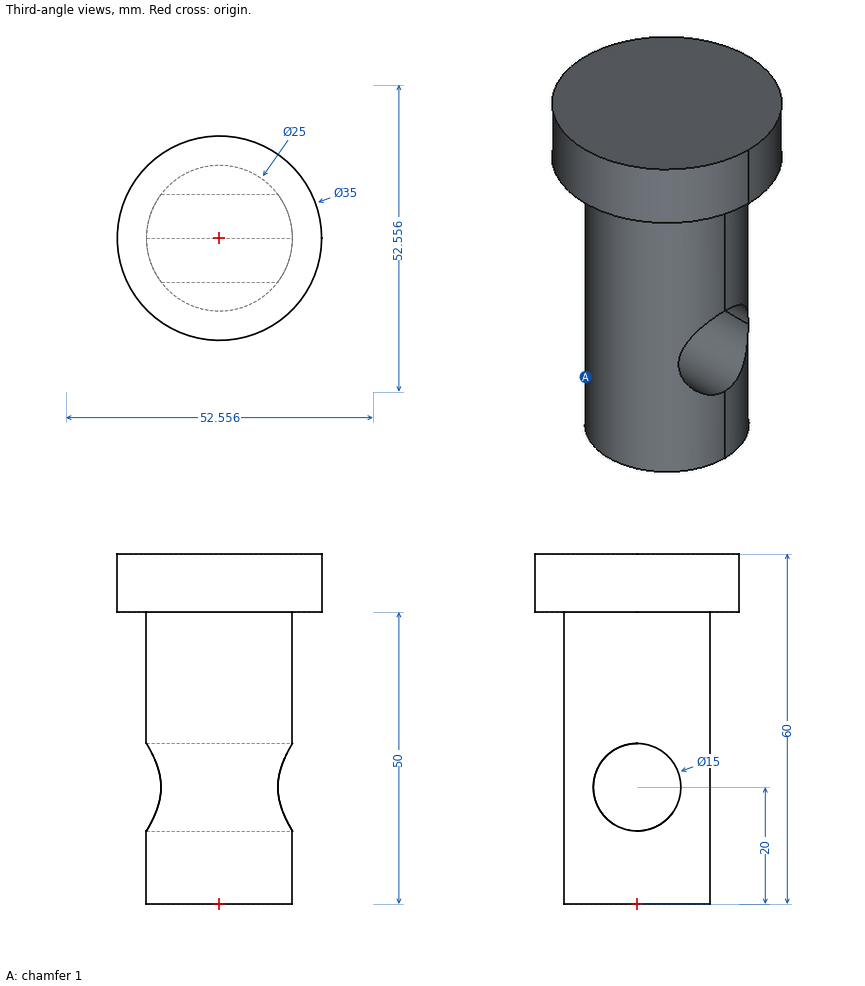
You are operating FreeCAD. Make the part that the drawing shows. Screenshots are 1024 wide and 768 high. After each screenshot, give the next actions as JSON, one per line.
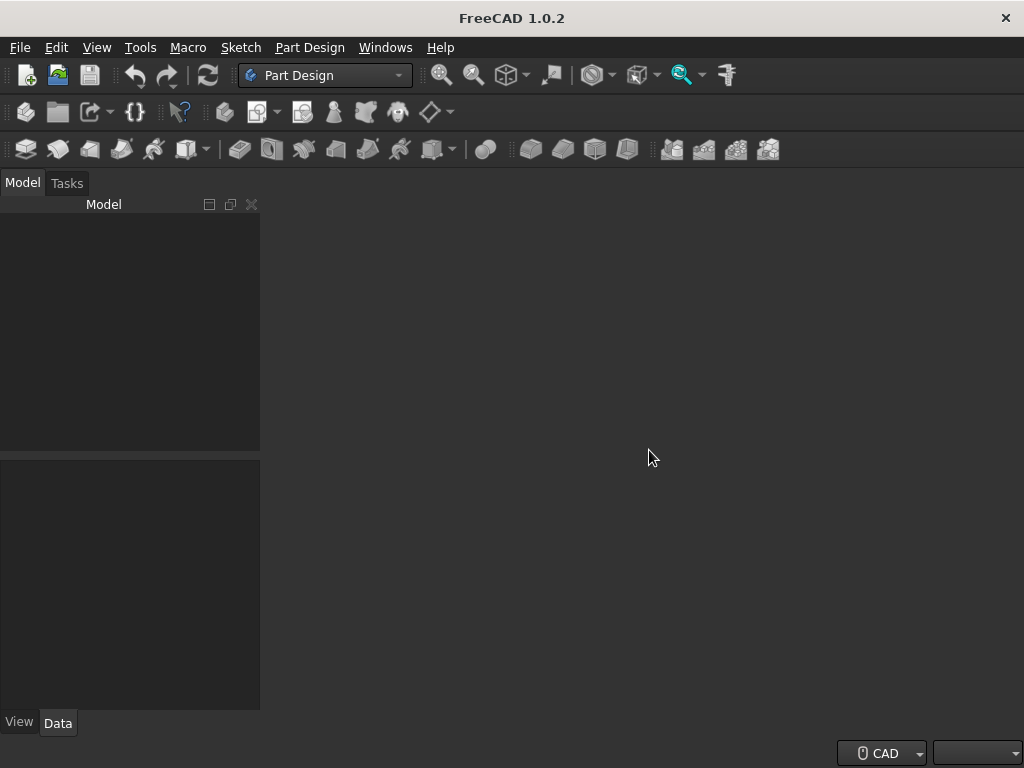
{"action": "key", "text": "ctrl+n"}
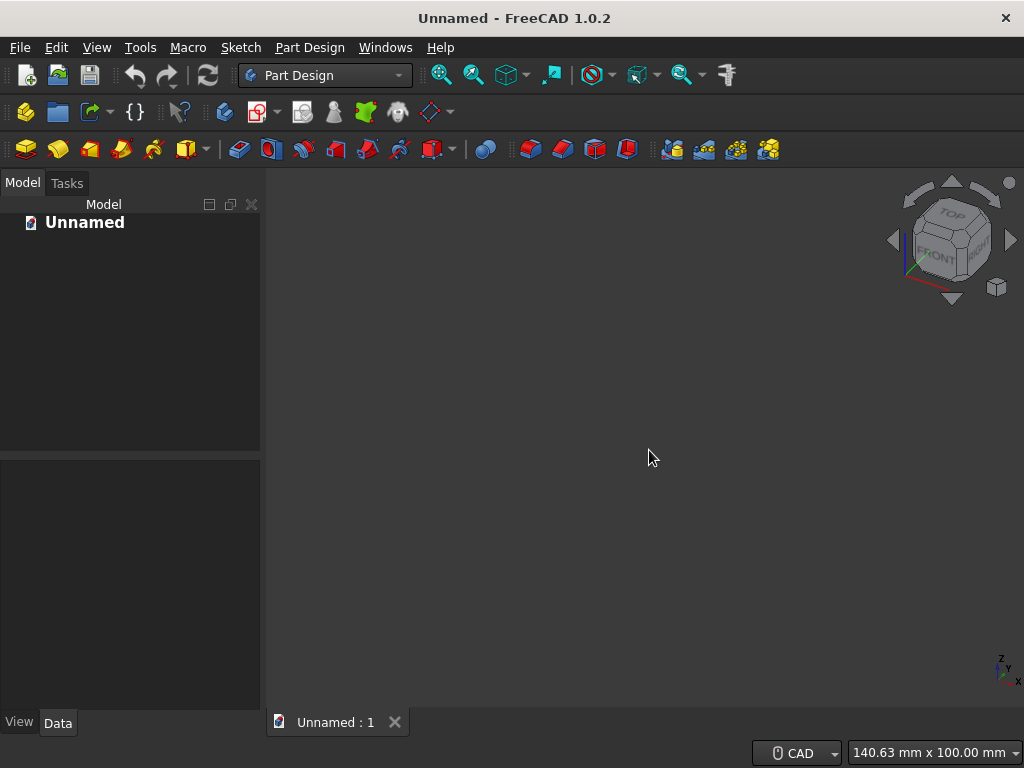
{"action": "left_click", "coordinate": [258, 112]}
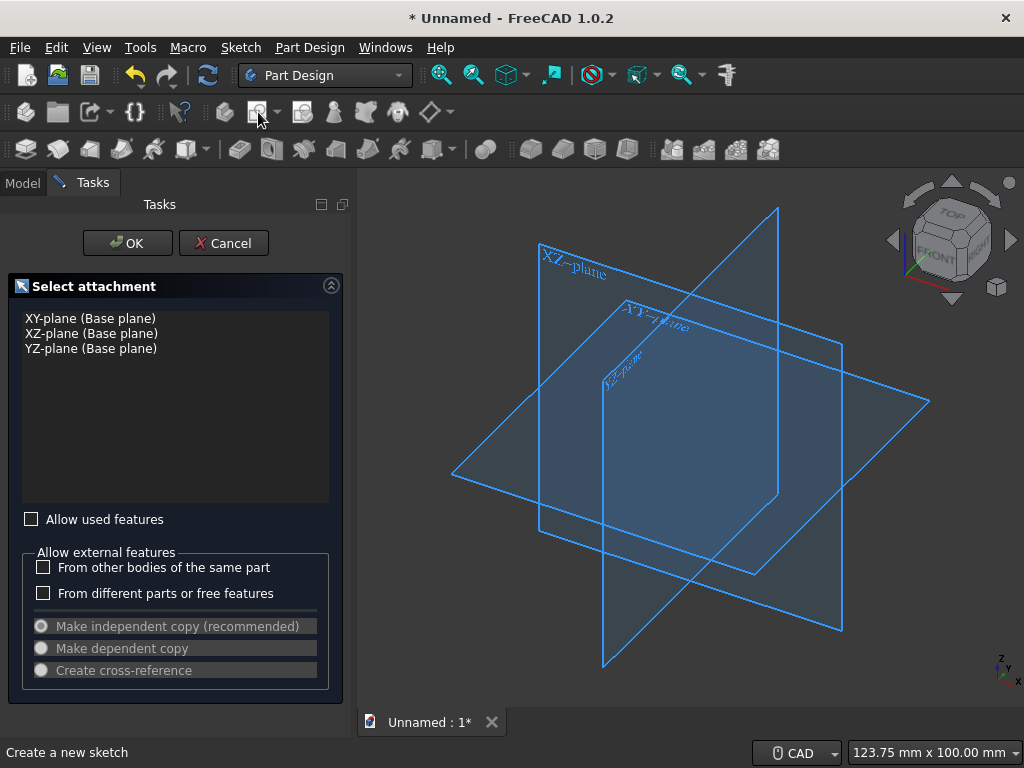
{"action": "left_click", "coordinate": [82, 318]}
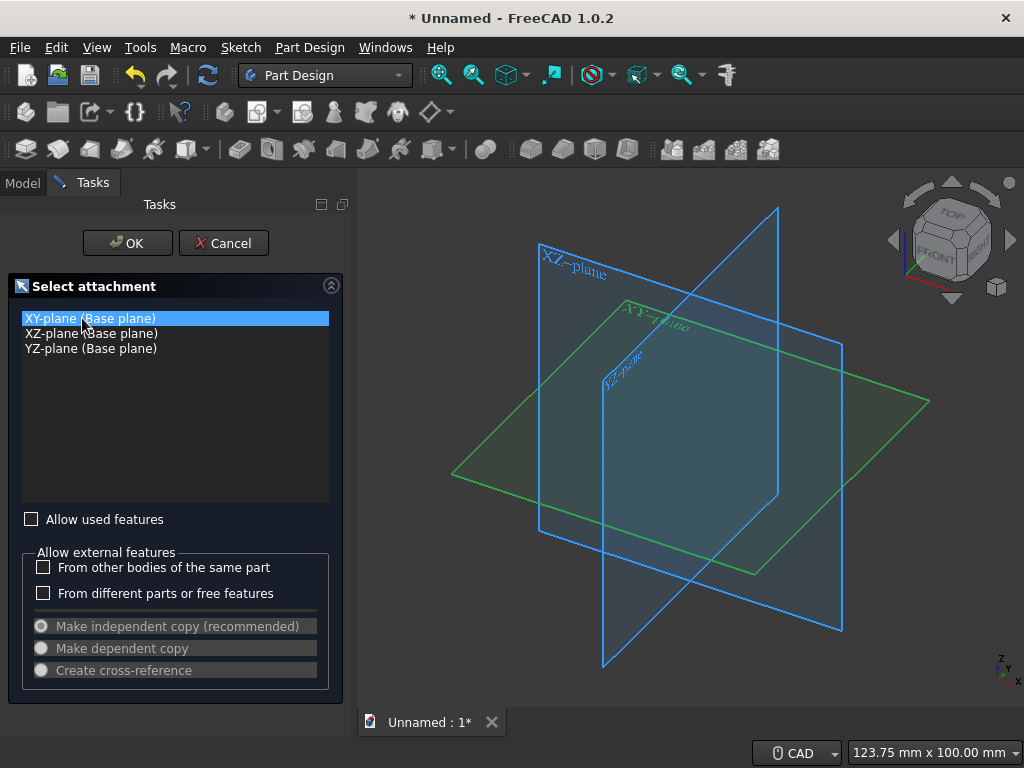
{"action": "left_click", "coordinate": [128, 243]}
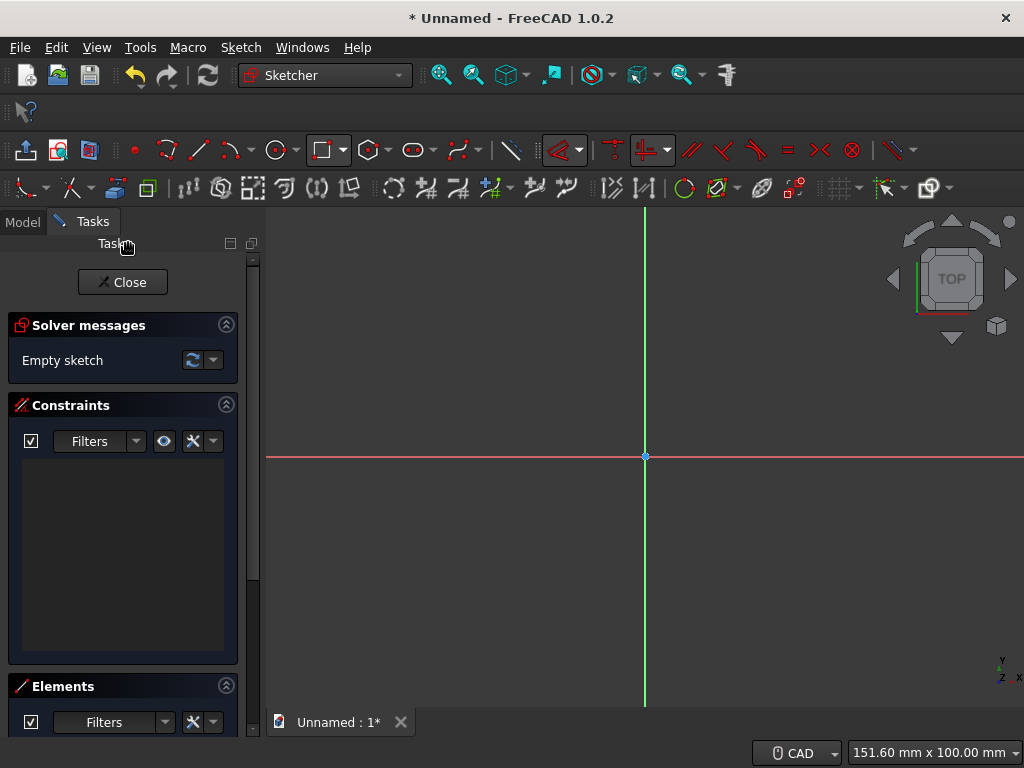
{"action": "scroll", "coordinate": [728, 457], "scroll_direction": "up", "scroll_amount": 3}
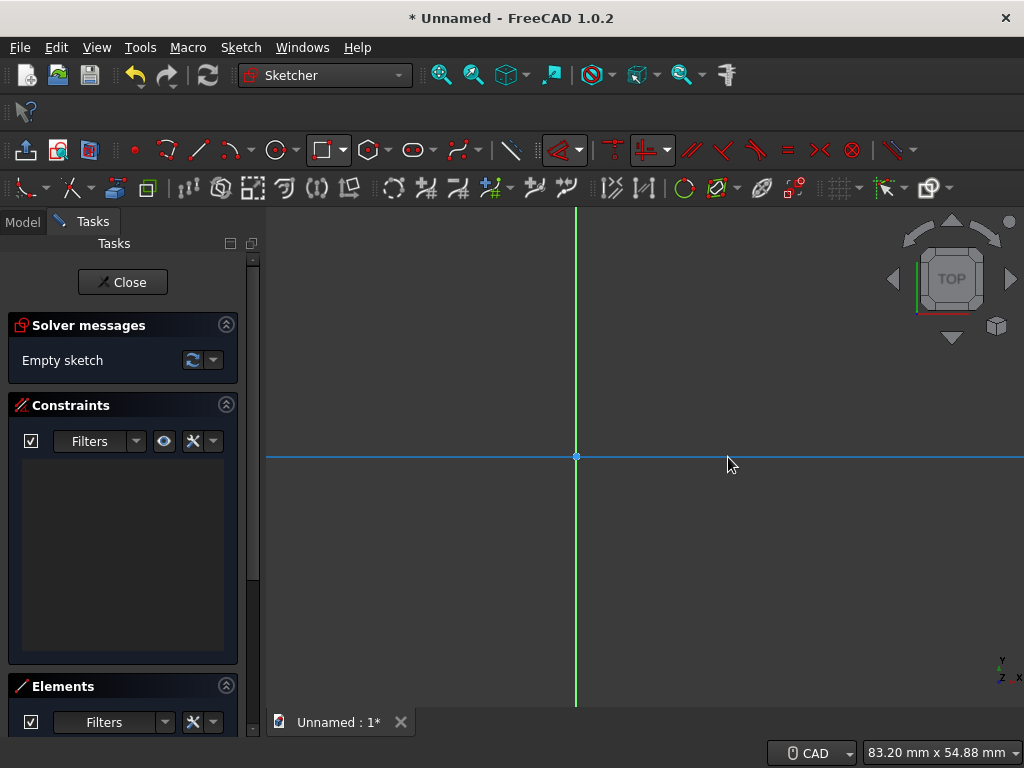
{"action": "left_click", "coordinate": [276, 150]}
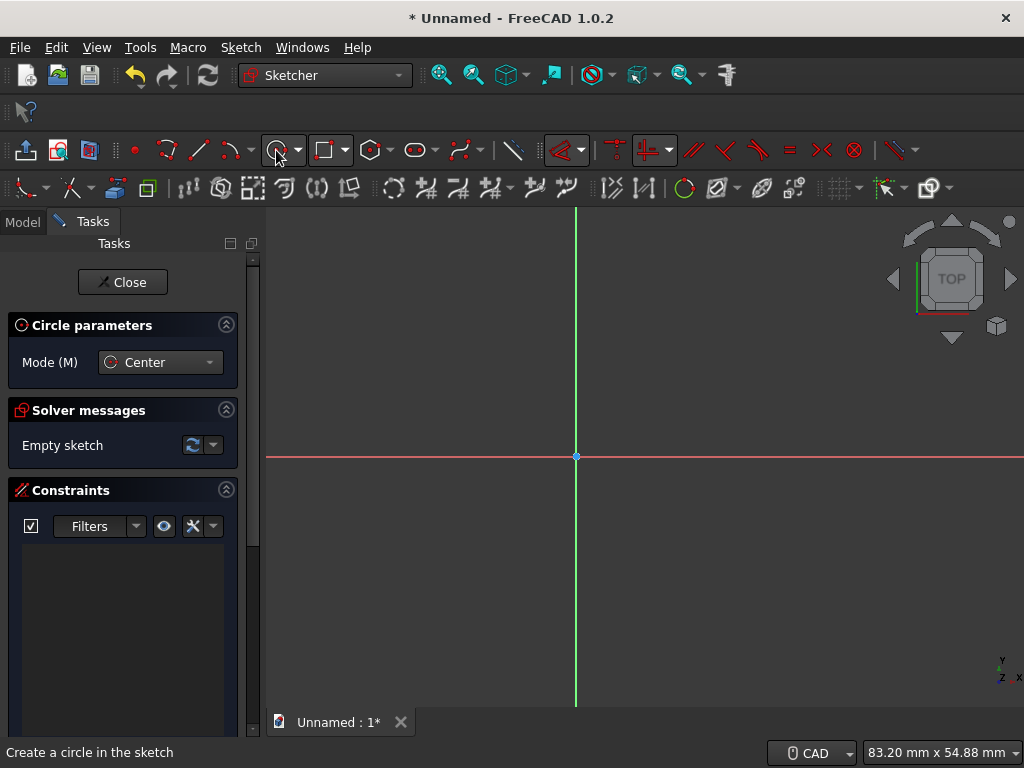
{"action": "left_click", "coordinate": [576, 457]}
{"action": "left_click", "coordinate": [689, 344]}
{"action": "key", "text": "Escape"}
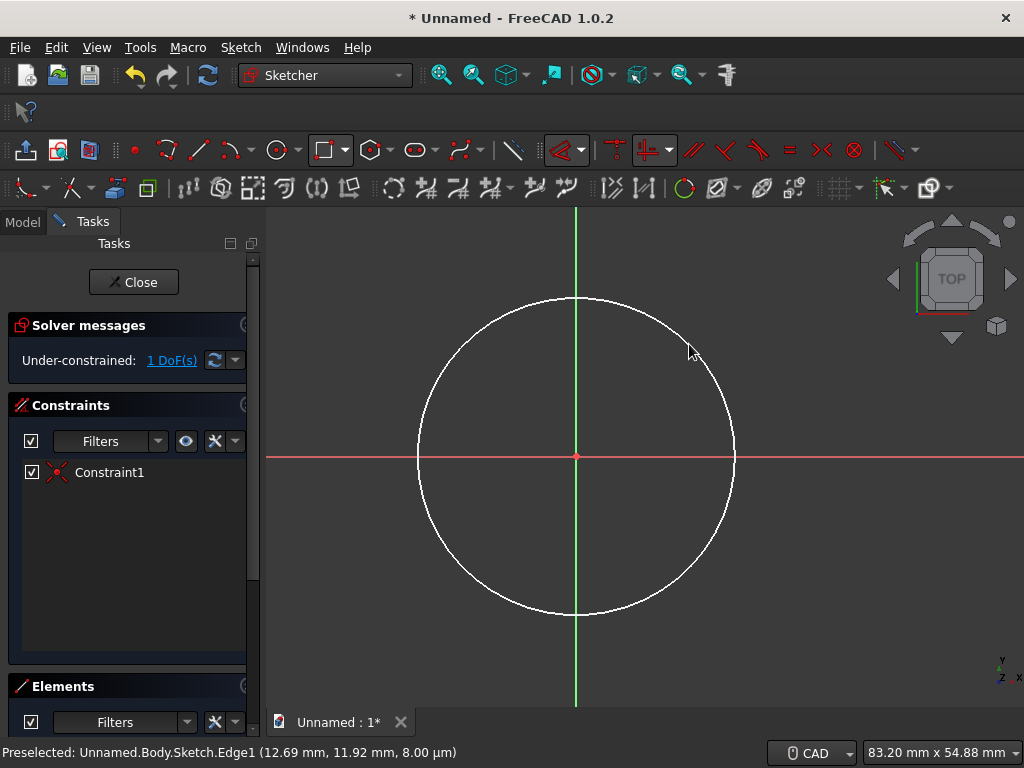
{"action": "left_click", "coordinate": [688, 344]}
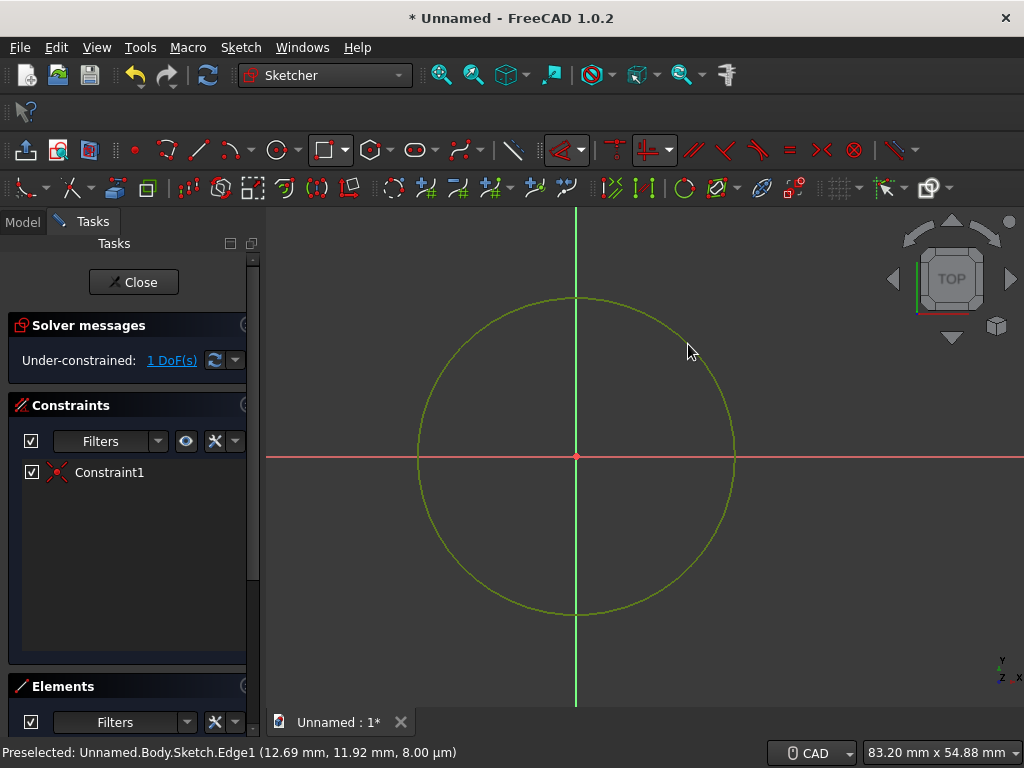
{"action": "left_click", "coordinate": [584, 150]}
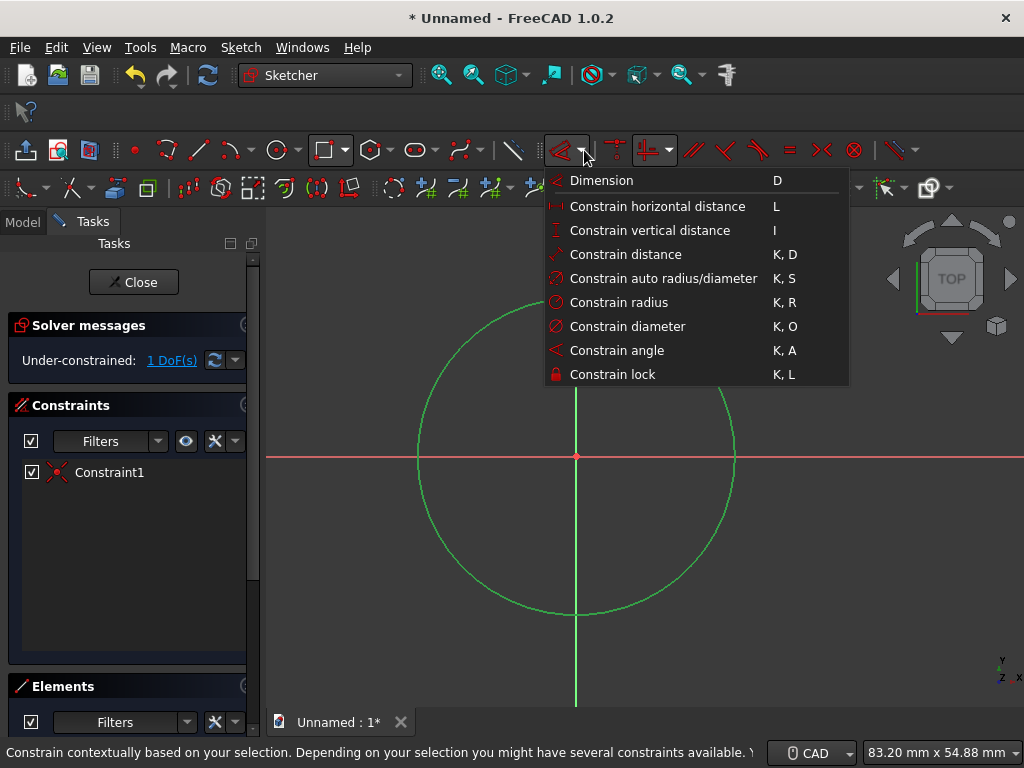
{"action": "left_click", "coordinate": [697, 326]}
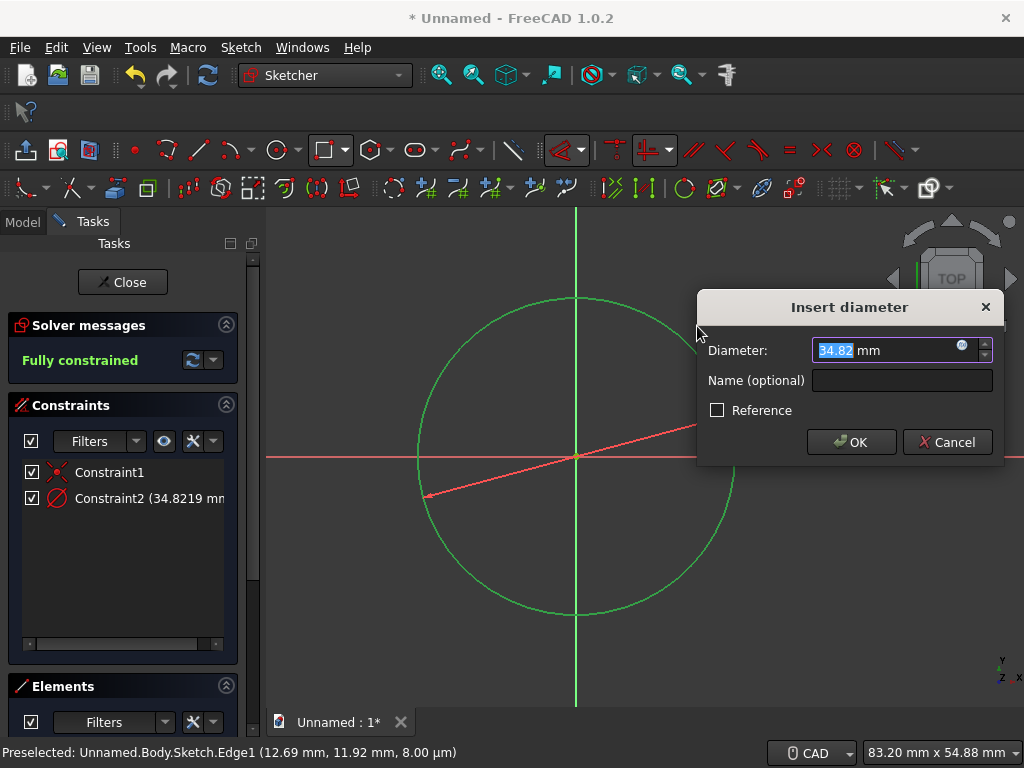
{"action": "type", "text": "35"}
{"action": "key", "text": "Return"}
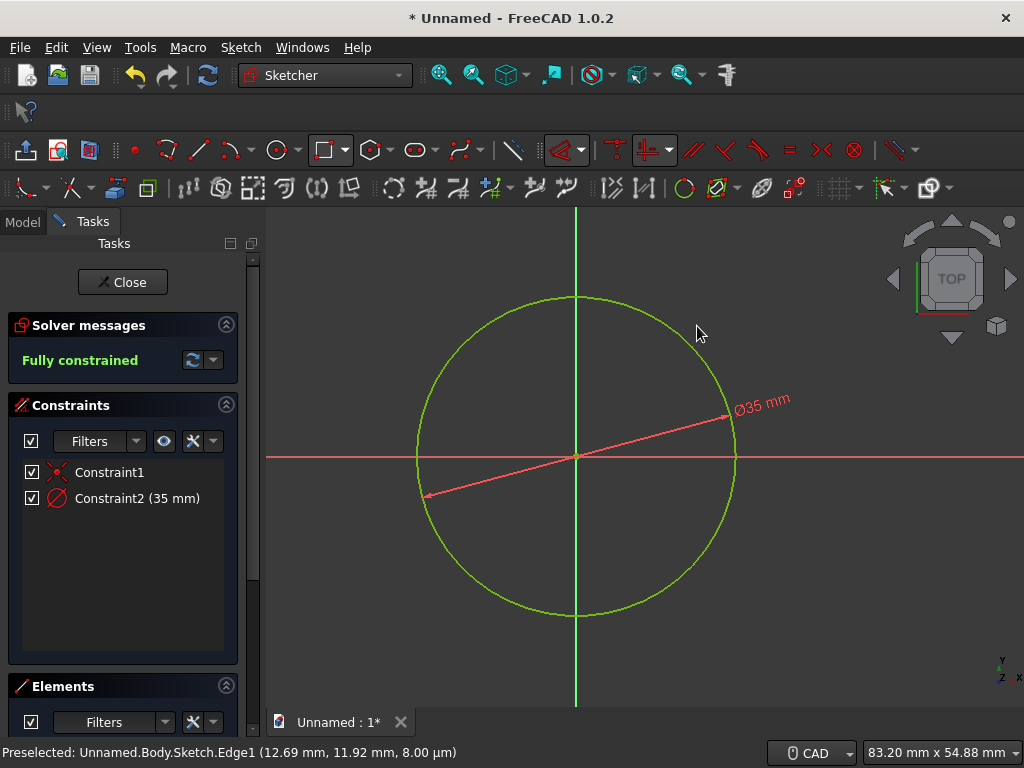
{"action": "left_click", "coordinate": [123, 282]}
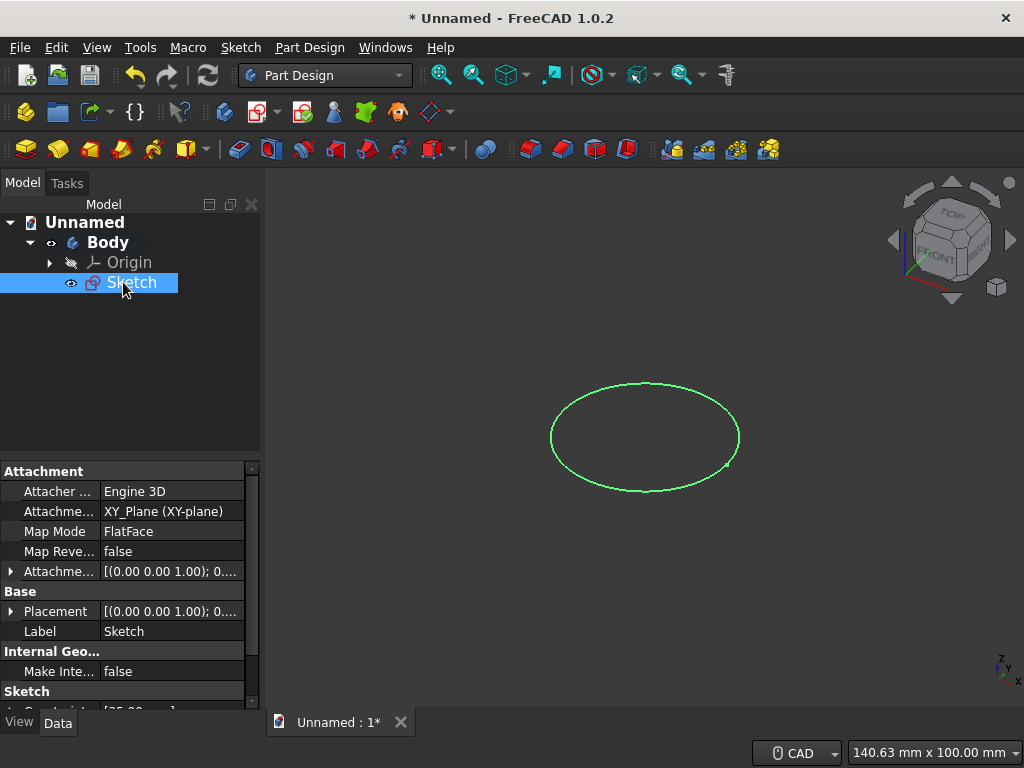
{"action": "left_click", "coordinate": [26, 150]}